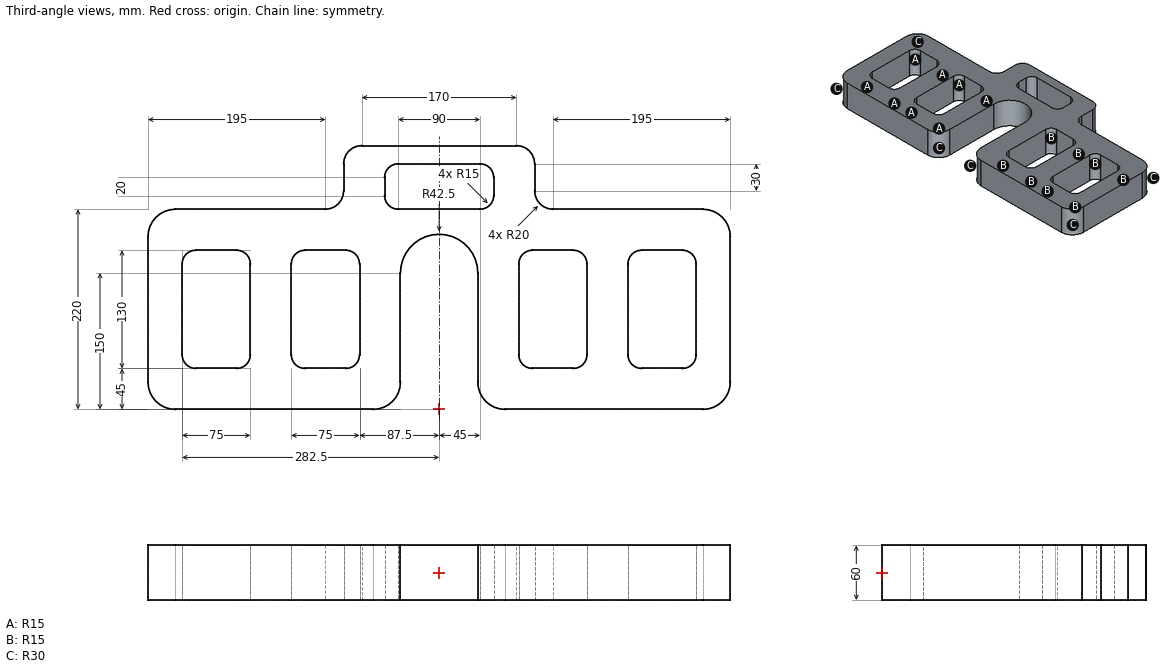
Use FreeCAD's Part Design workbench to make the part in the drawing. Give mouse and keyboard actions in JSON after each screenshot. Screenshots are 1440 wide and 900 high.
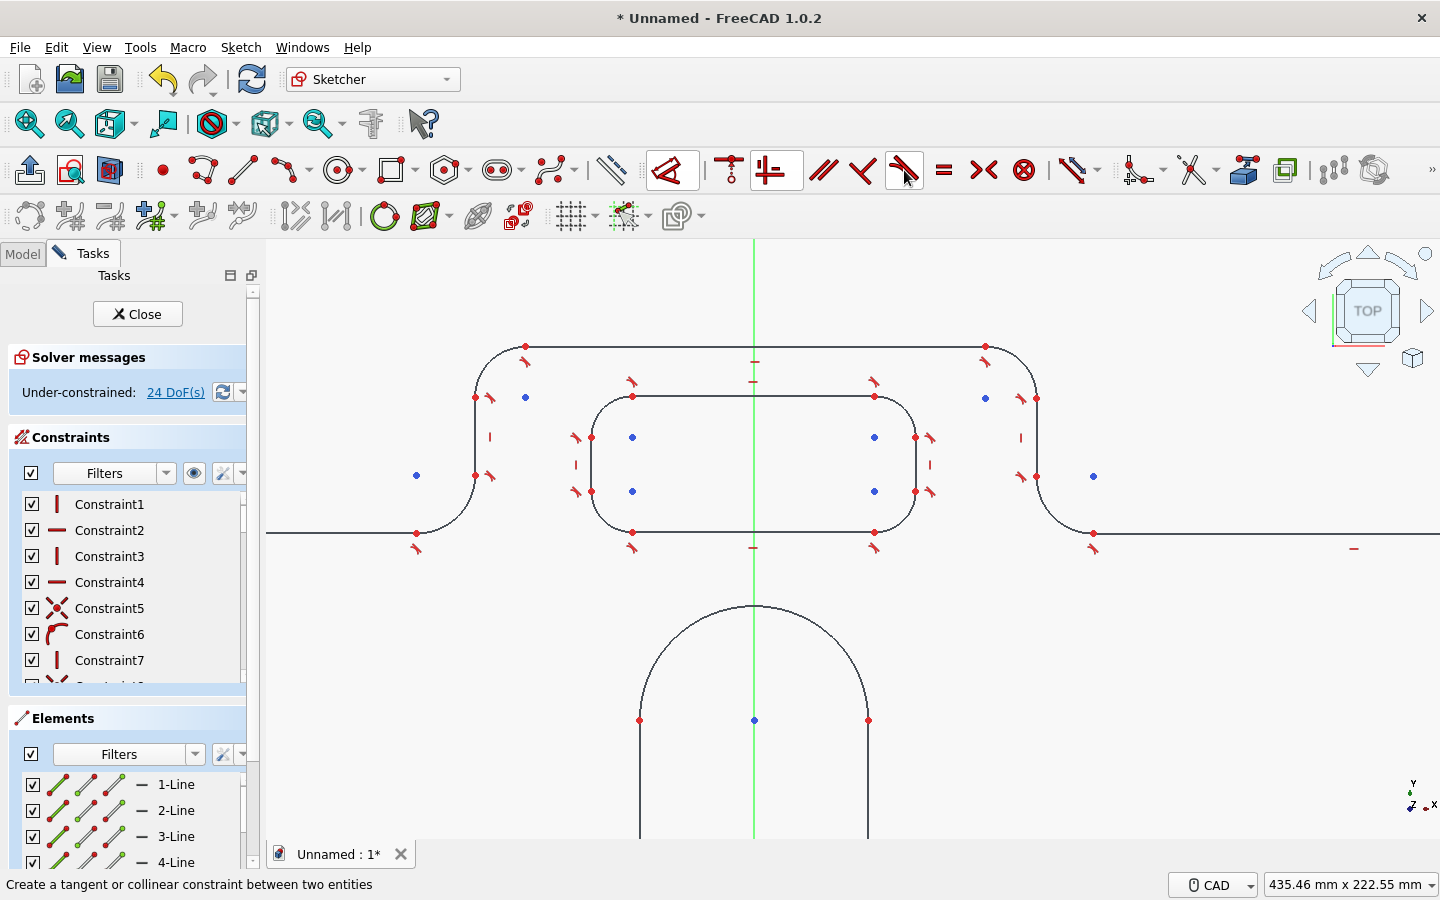
{"action": "left_click", "coordinate": [1031, 375]}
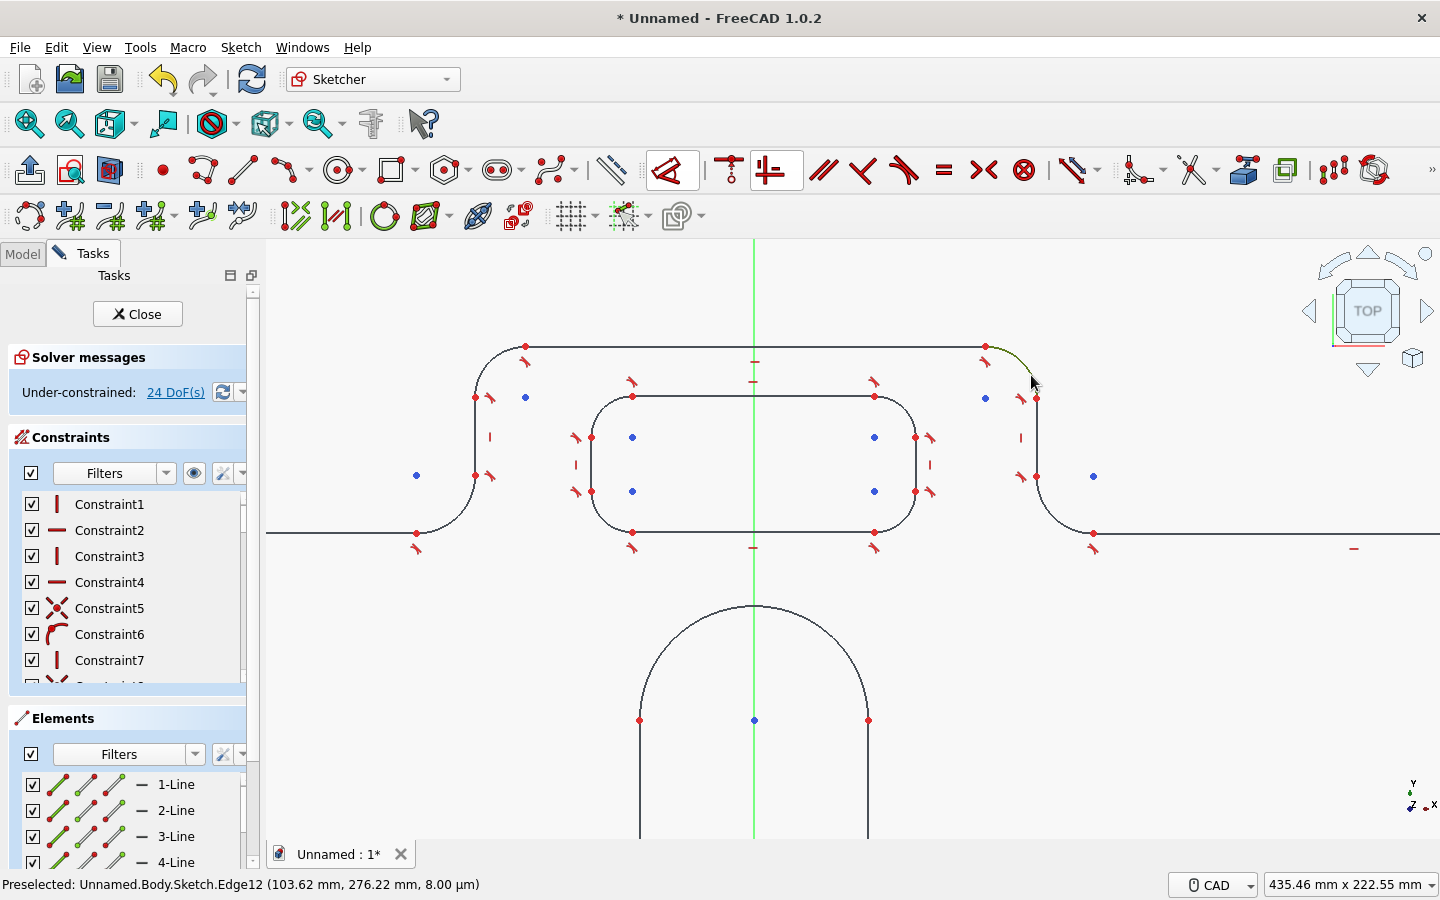
{"action": "left_click", "coordinate": [503, 352]}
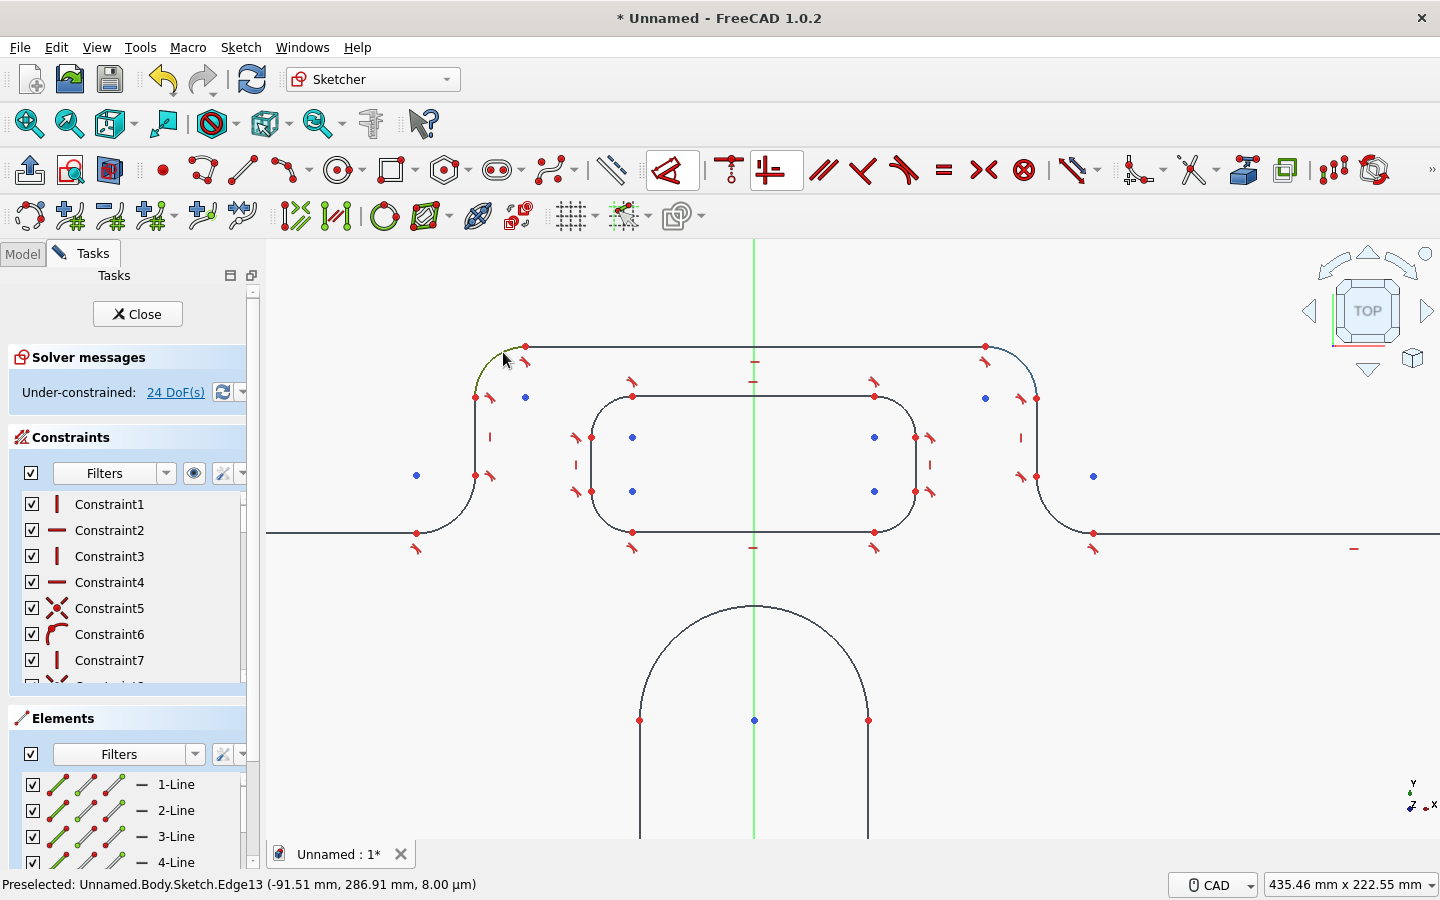
{"action": "left_click", "coordinate": [443, 527]}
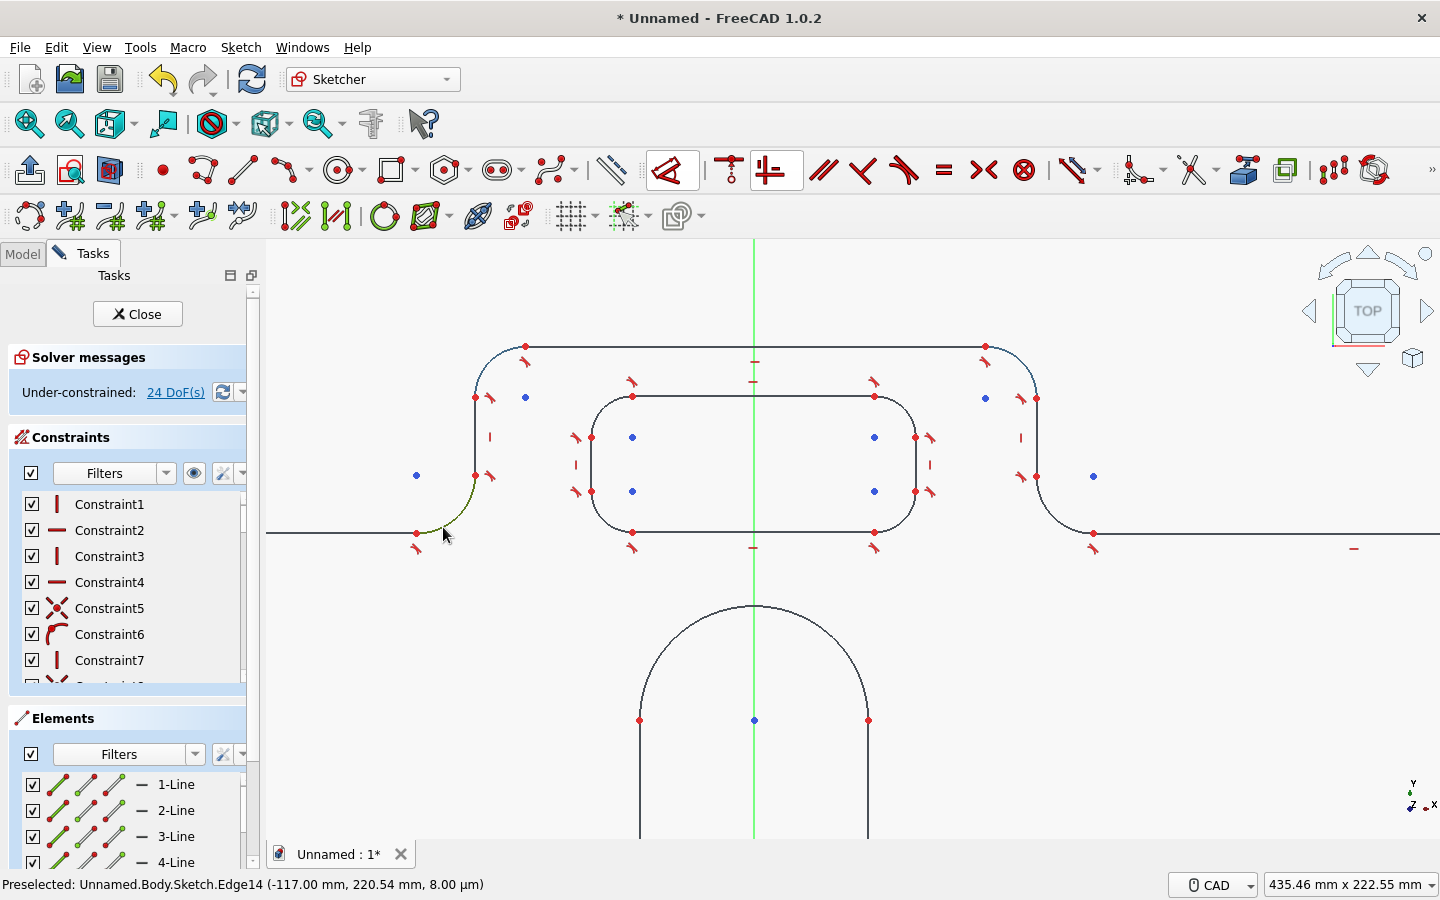
{"action": "left_click", "coordinate": [1043, 503]}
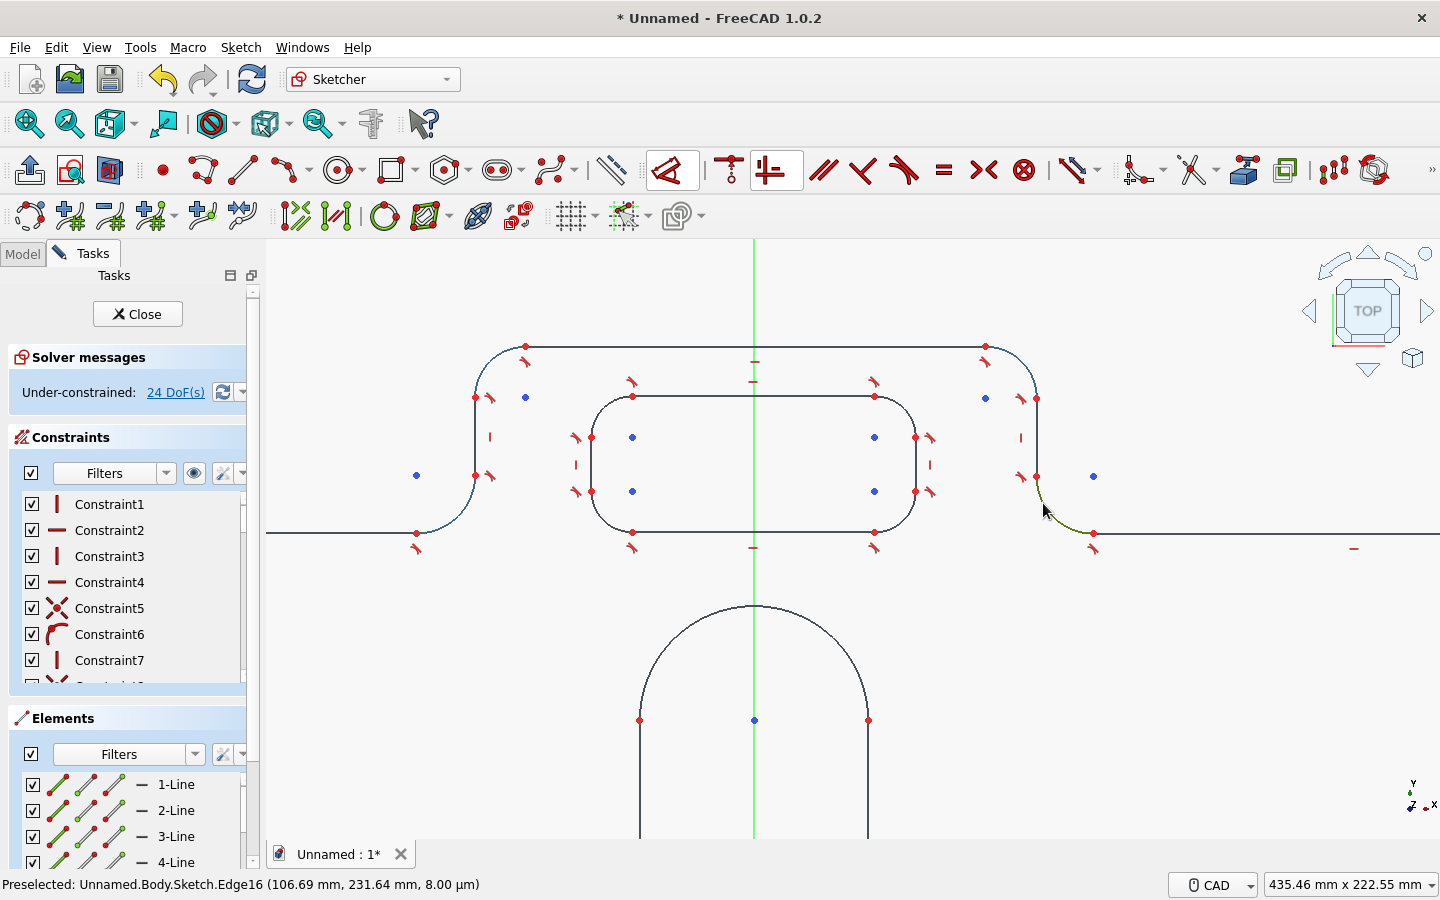
{"action": "left_click", "coordinate": [944, 170]}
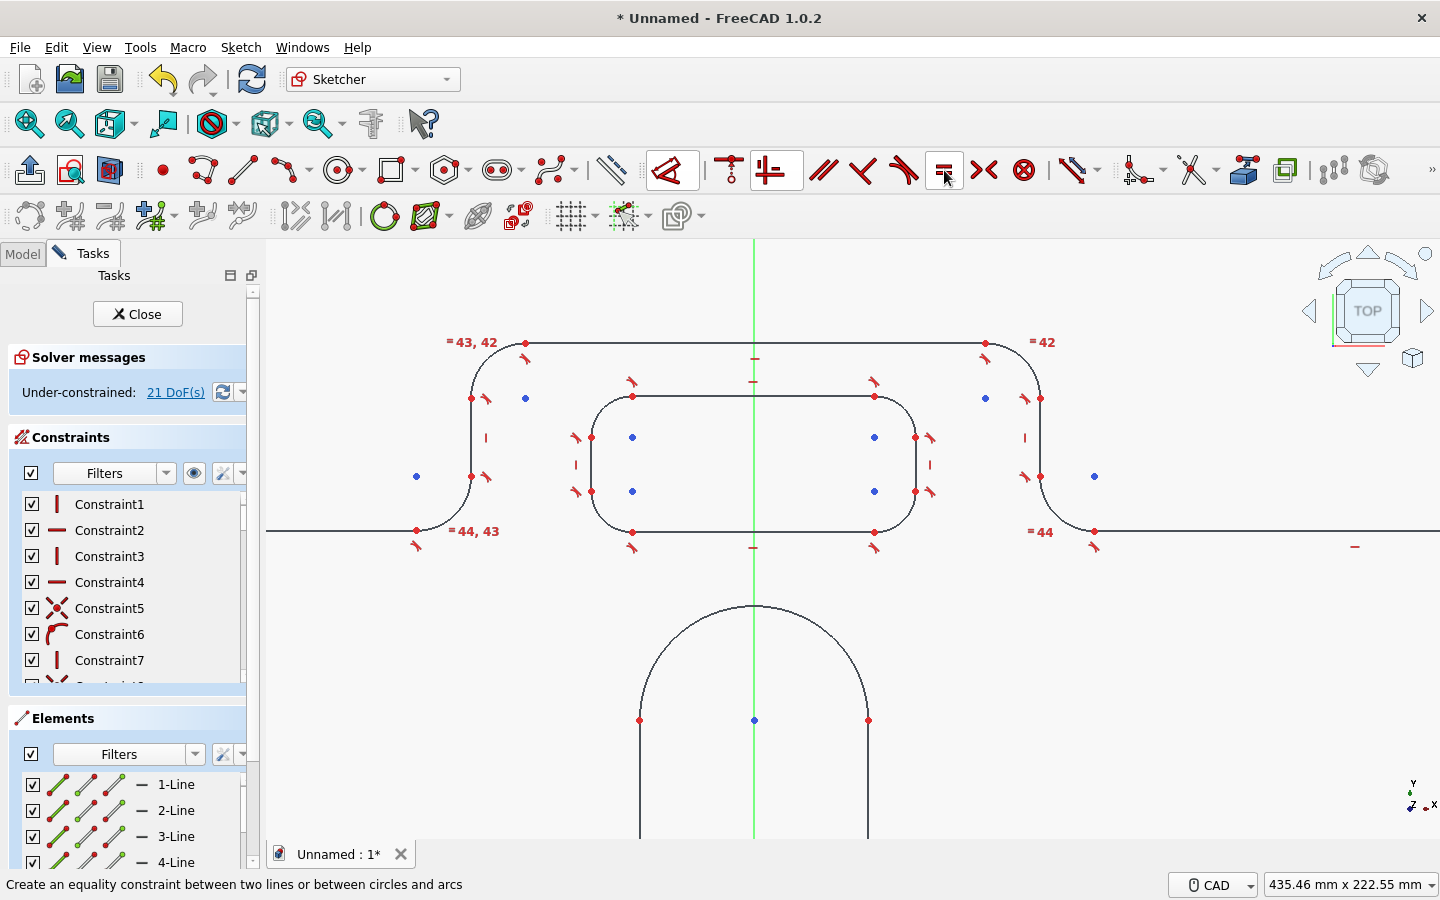
{"action": "left_click", "coordinate": [596, 510]}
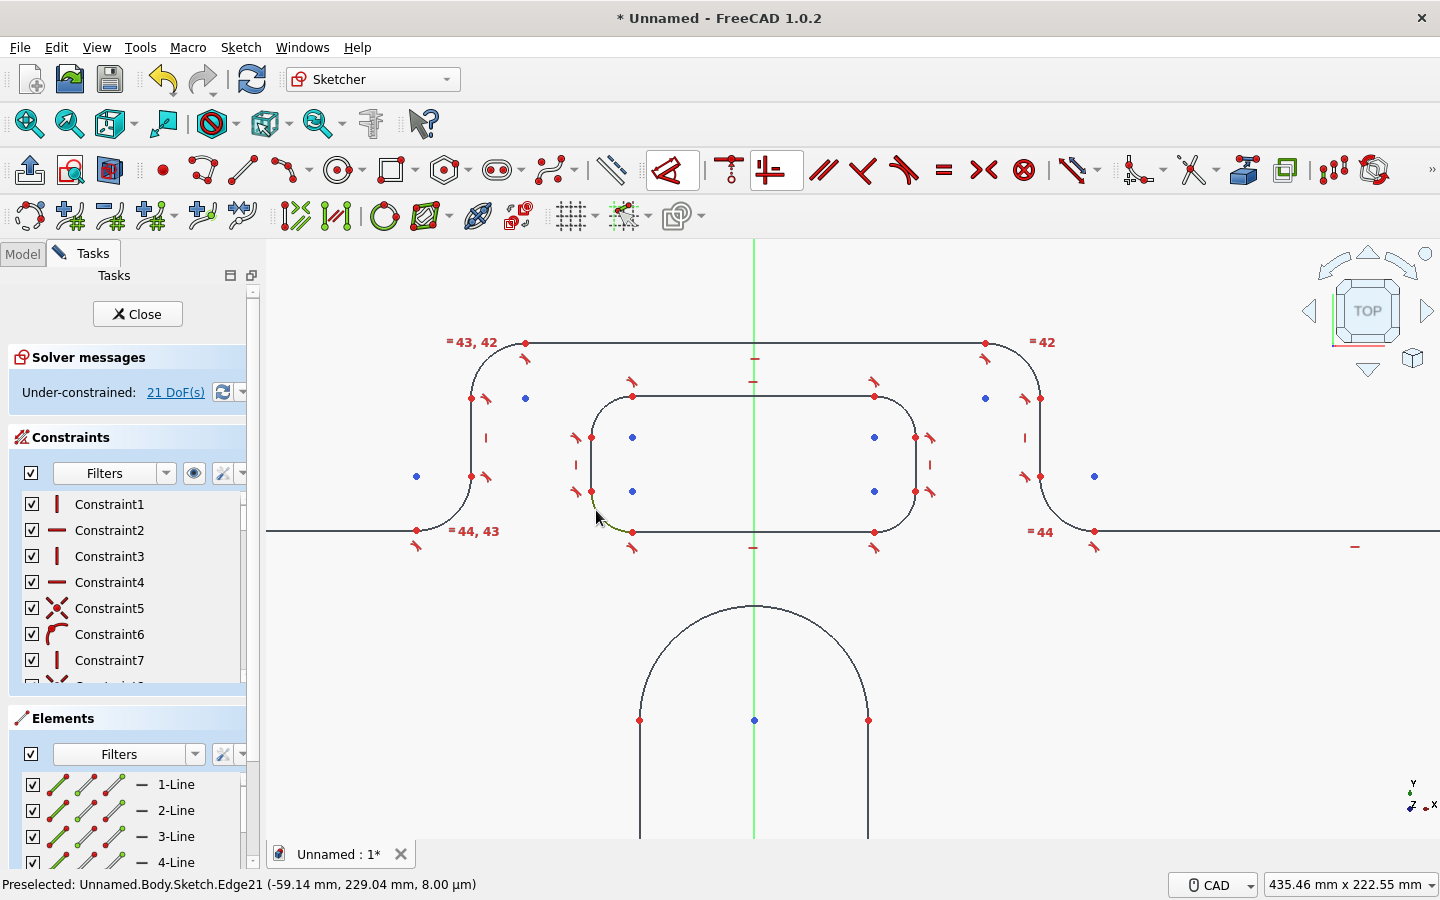
{"action": "left_click", "coordinate": [614, 401]}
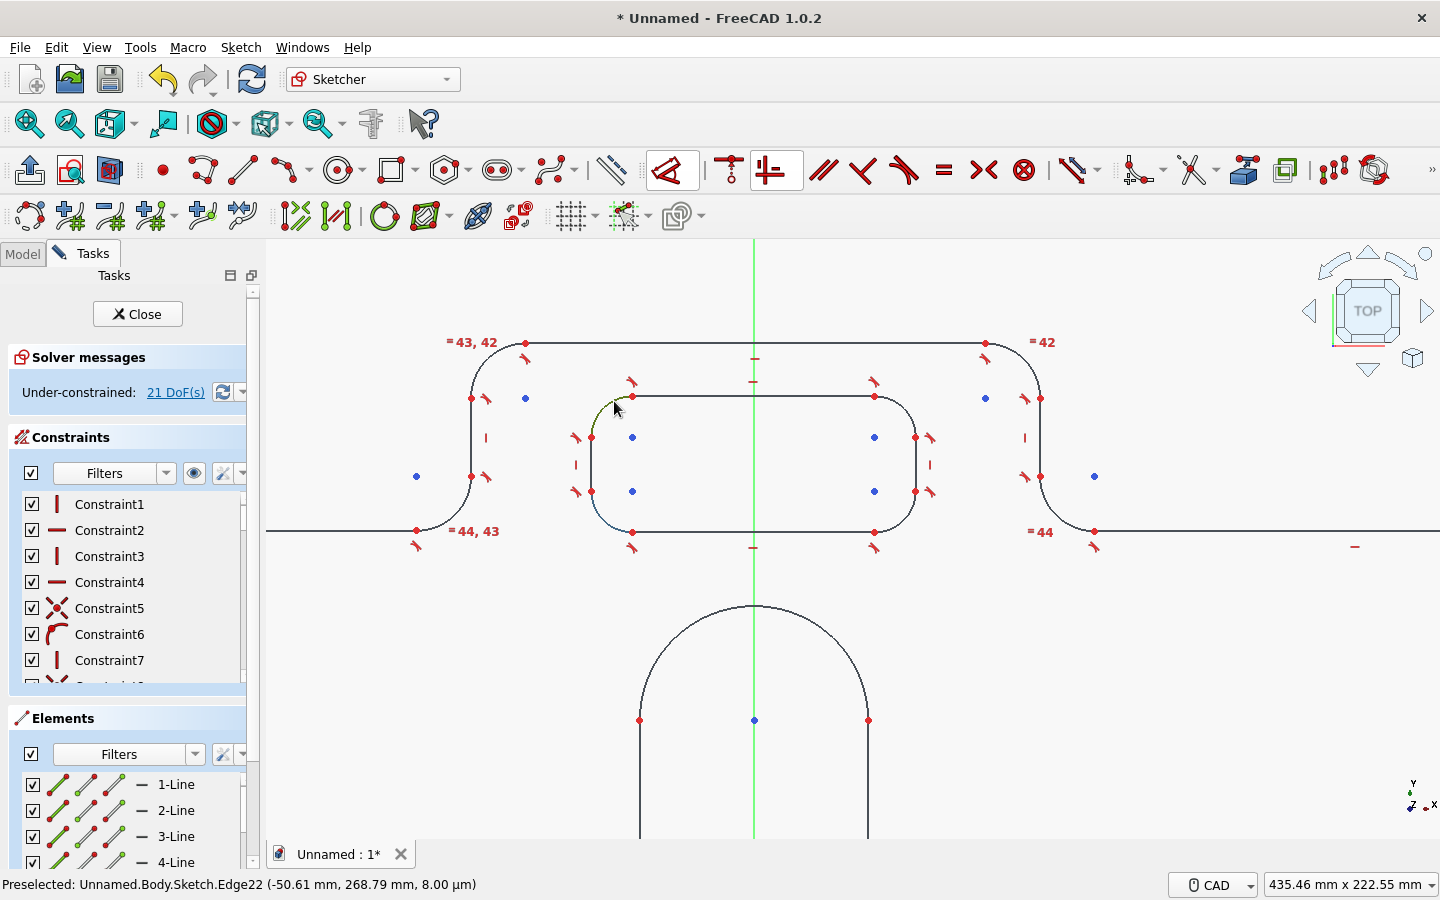
{"action": "left_click", "coordinate": [911, 419]}